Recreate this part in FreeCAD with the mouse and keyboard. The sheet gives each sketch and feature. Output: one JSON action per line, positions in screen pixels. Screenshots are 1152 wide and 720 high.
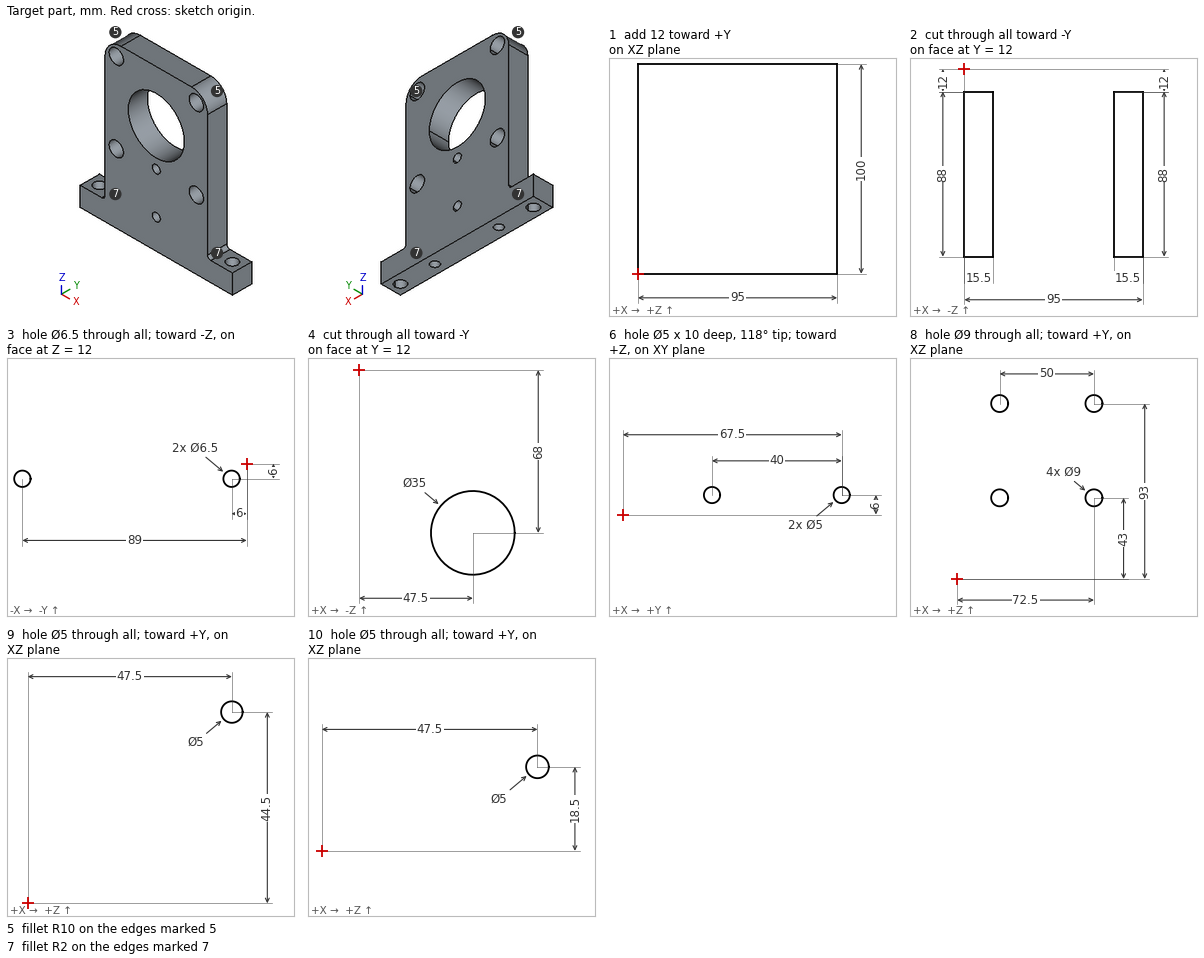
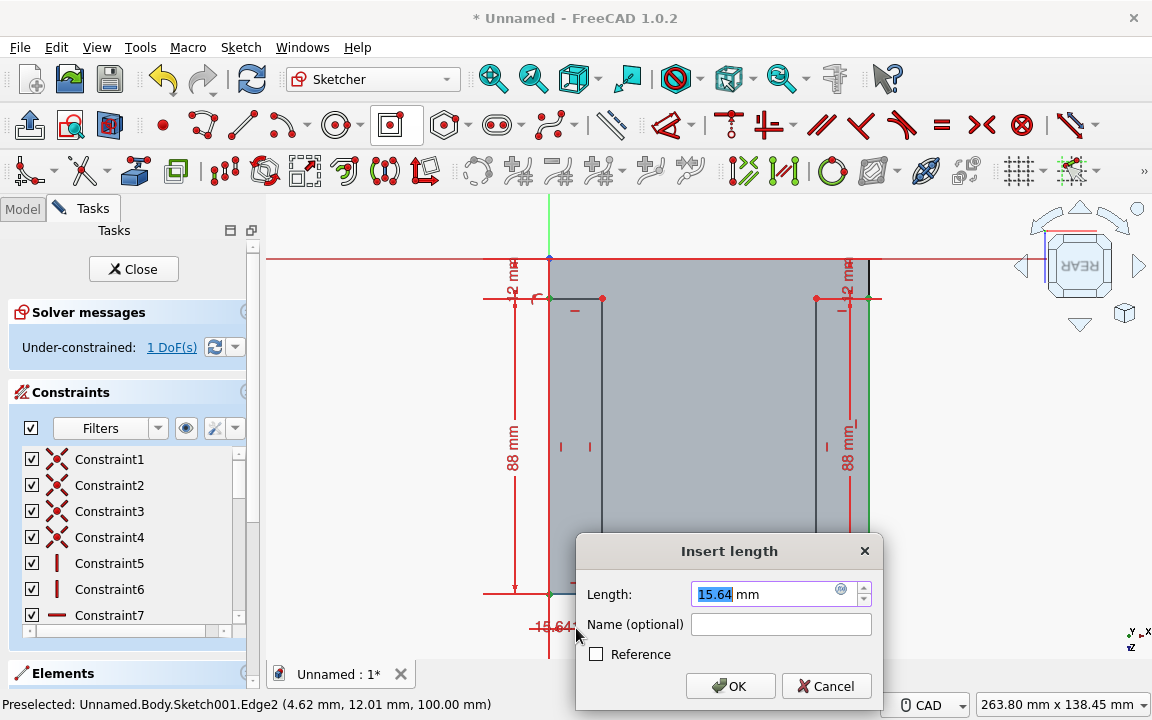
{"action": "type", "text": "15.5"}
{"action": "key", "text": "Return"}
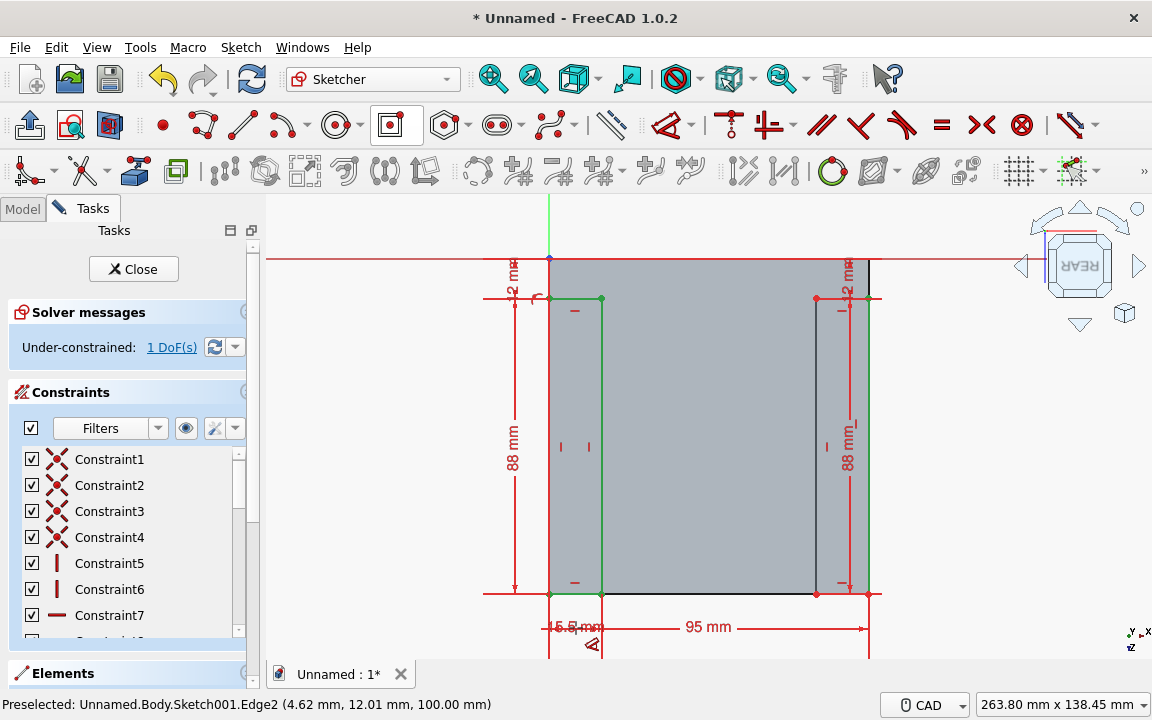
{"action": "left_click", "coordinate": [832, 594]}
{"action": "left_click", "coordinate": [842, 628]}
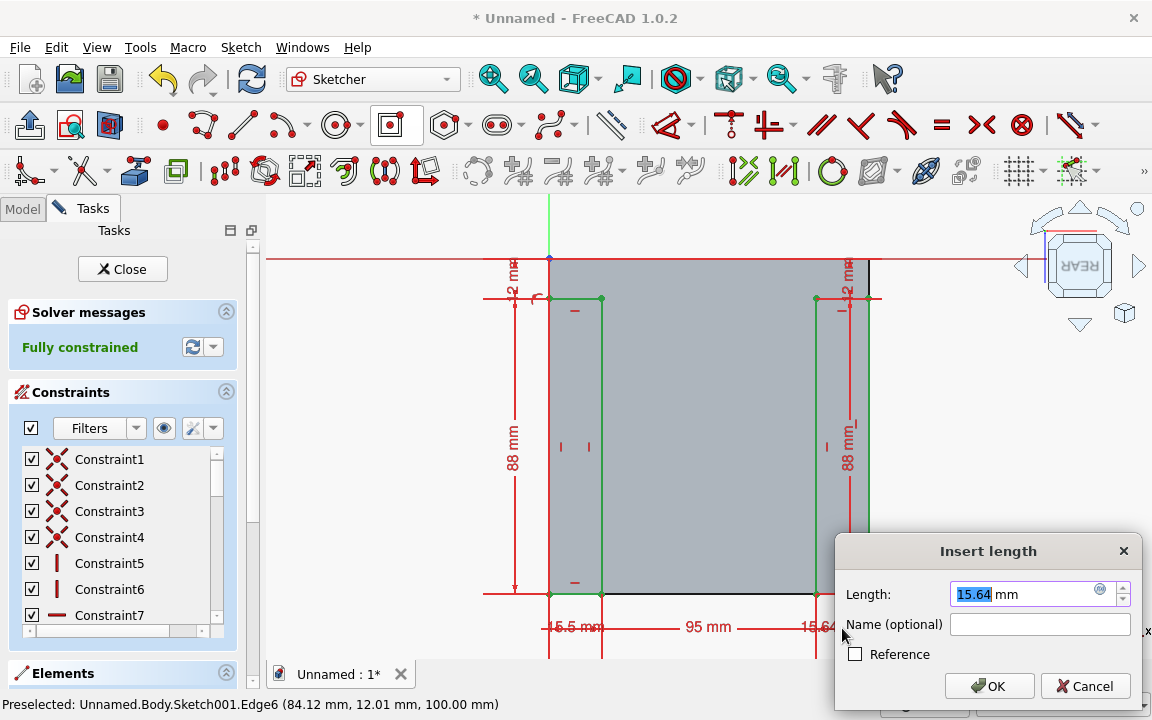
{"action": "type", "text": "15.5"}
{"action": "key", "text": "Return"}
{"action": "key", "text": "Escape"}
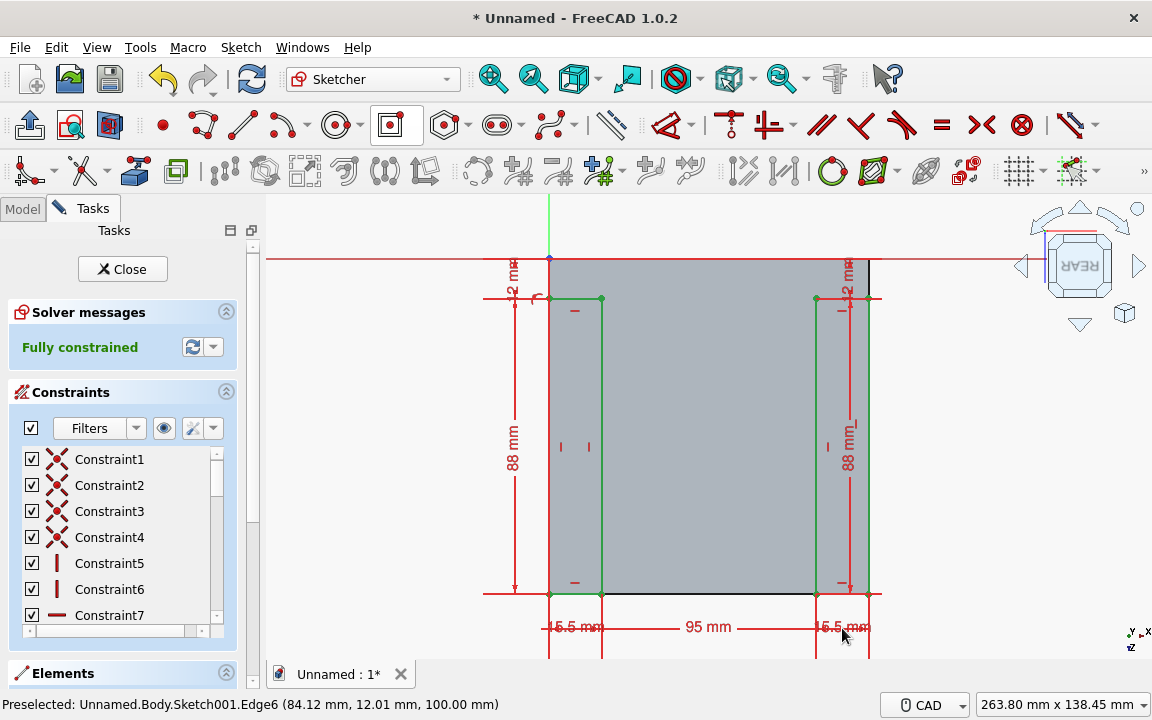
{"action": "left_click", "coordinate": [123, 269]}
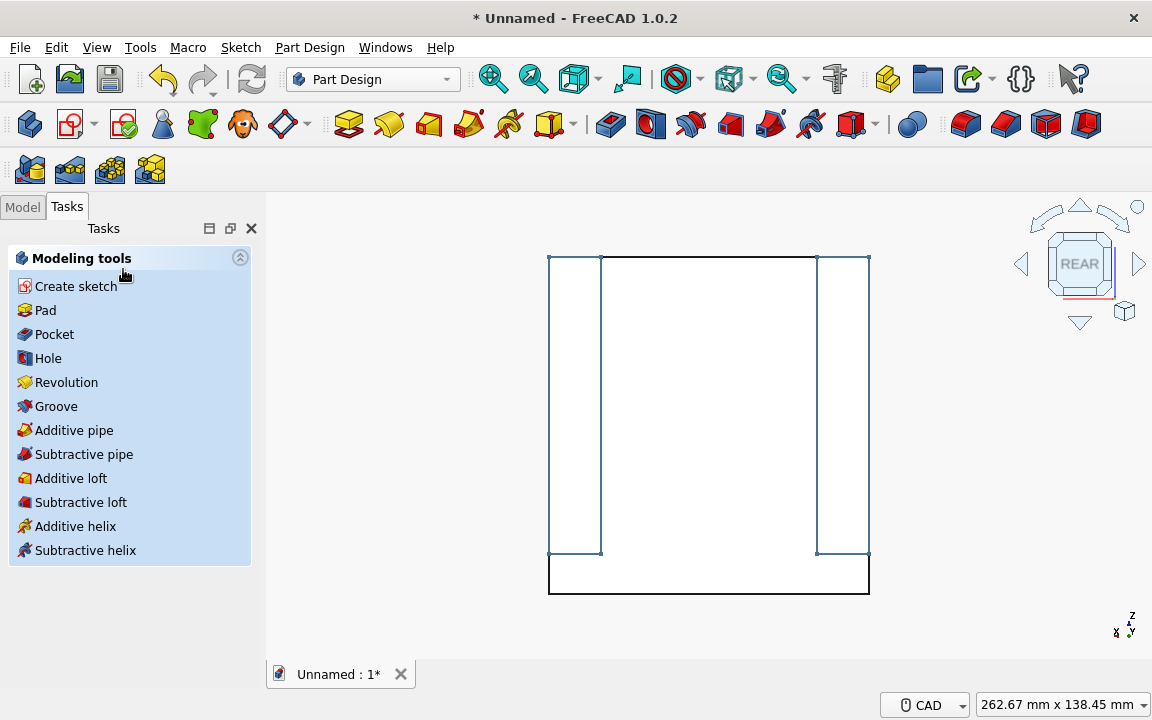
{"action": "left_click", "coordinate": [612, 124]}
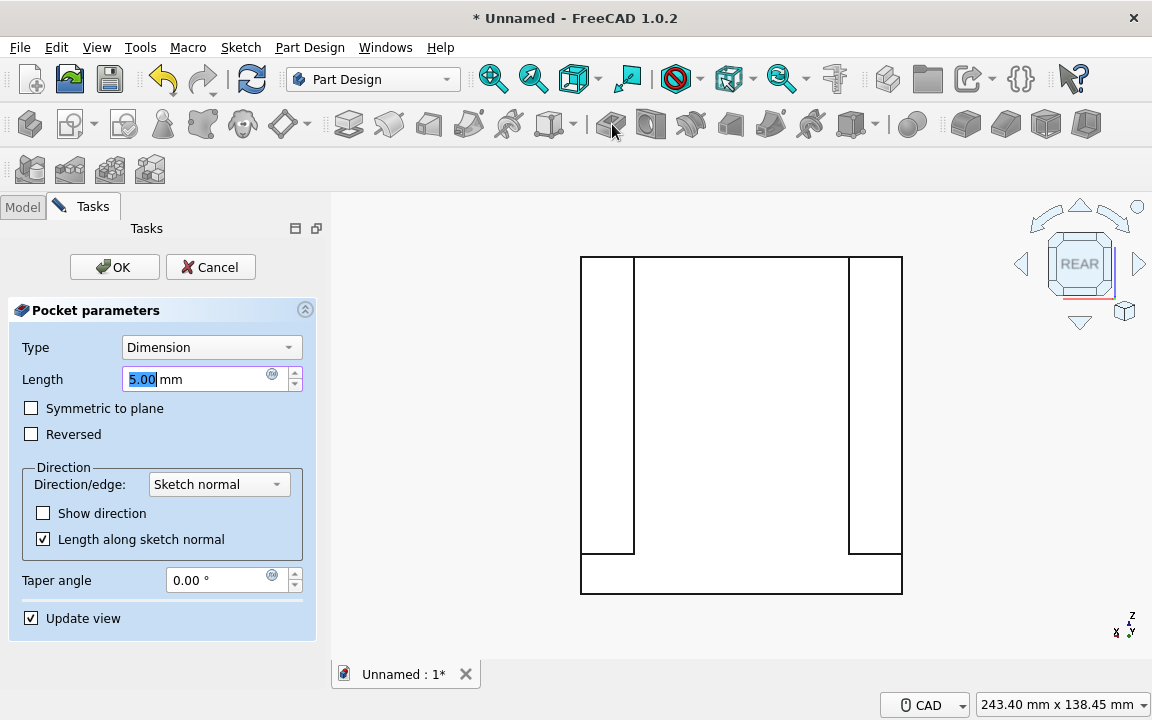
{"action": "left_click", "coordinate": [212, 348]}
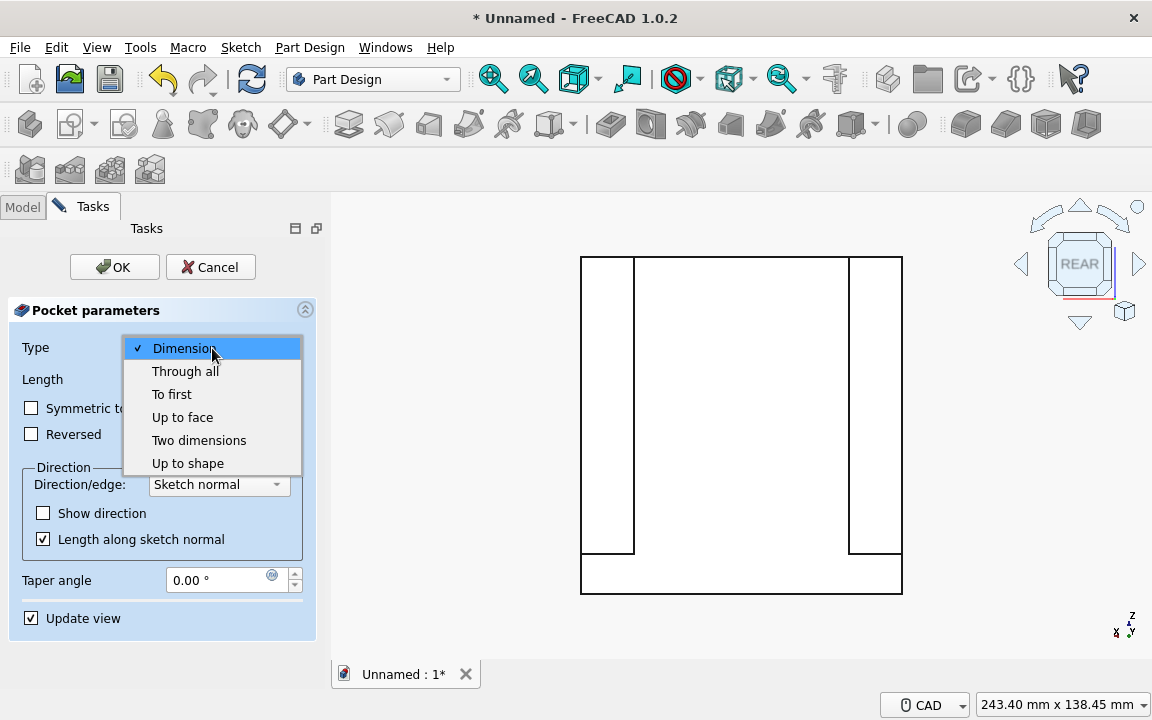
{"action": "left_click", "coordinate": [212, 372]}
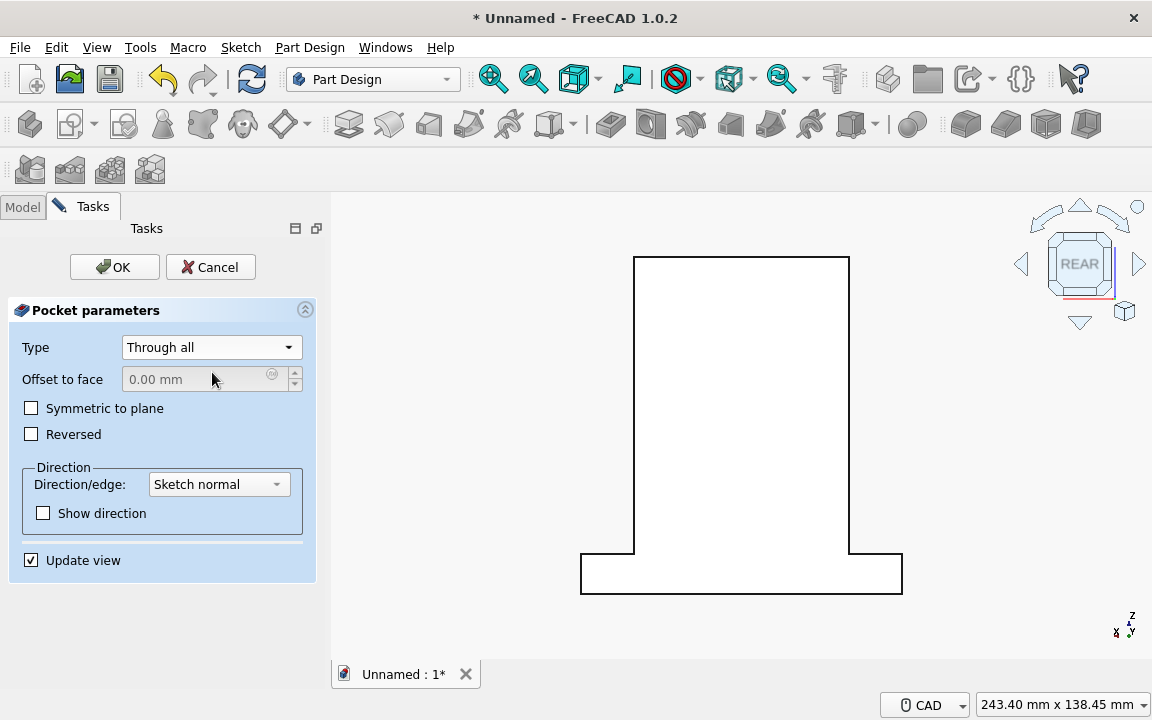
{"action": "left_click", "coordinate": [115, 267]}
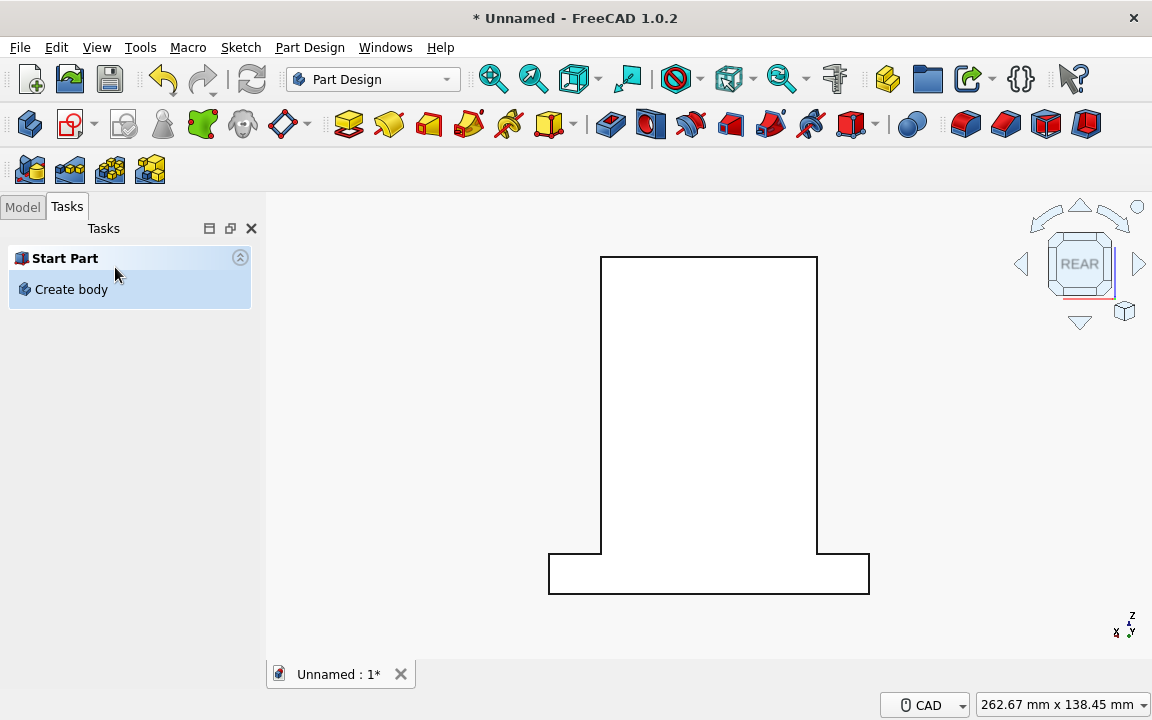
{"action": "key", "text": "0"}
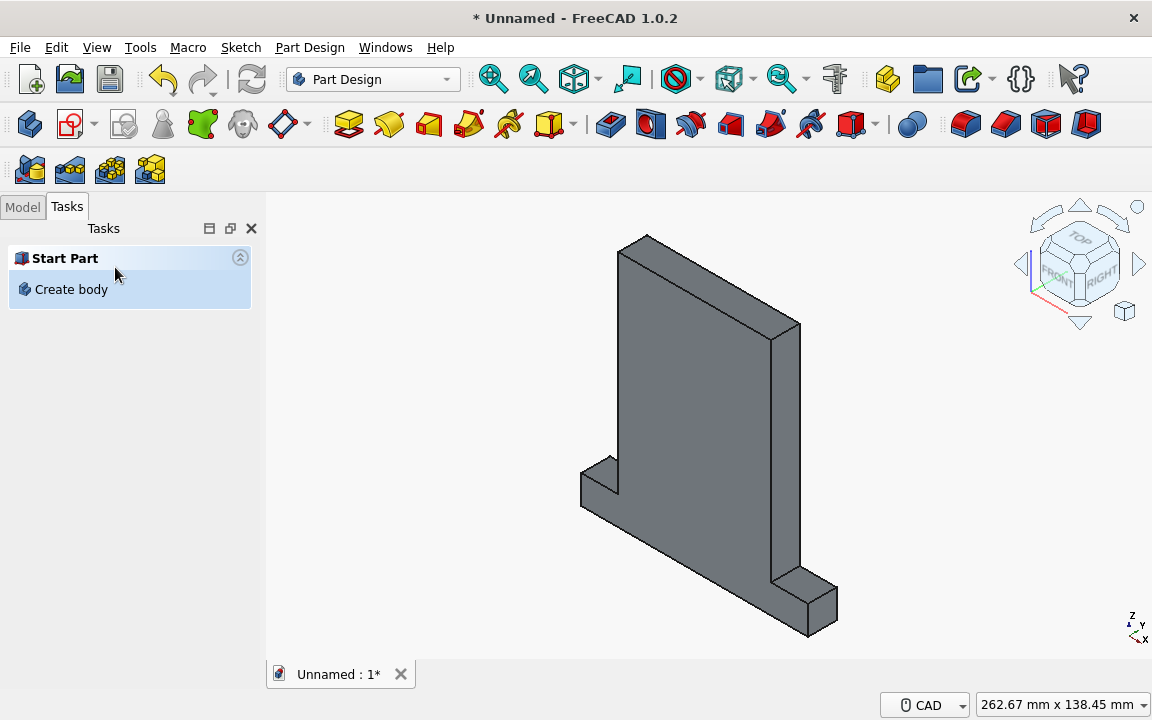
{"action": "left_click", "coordinate": [609, 471]}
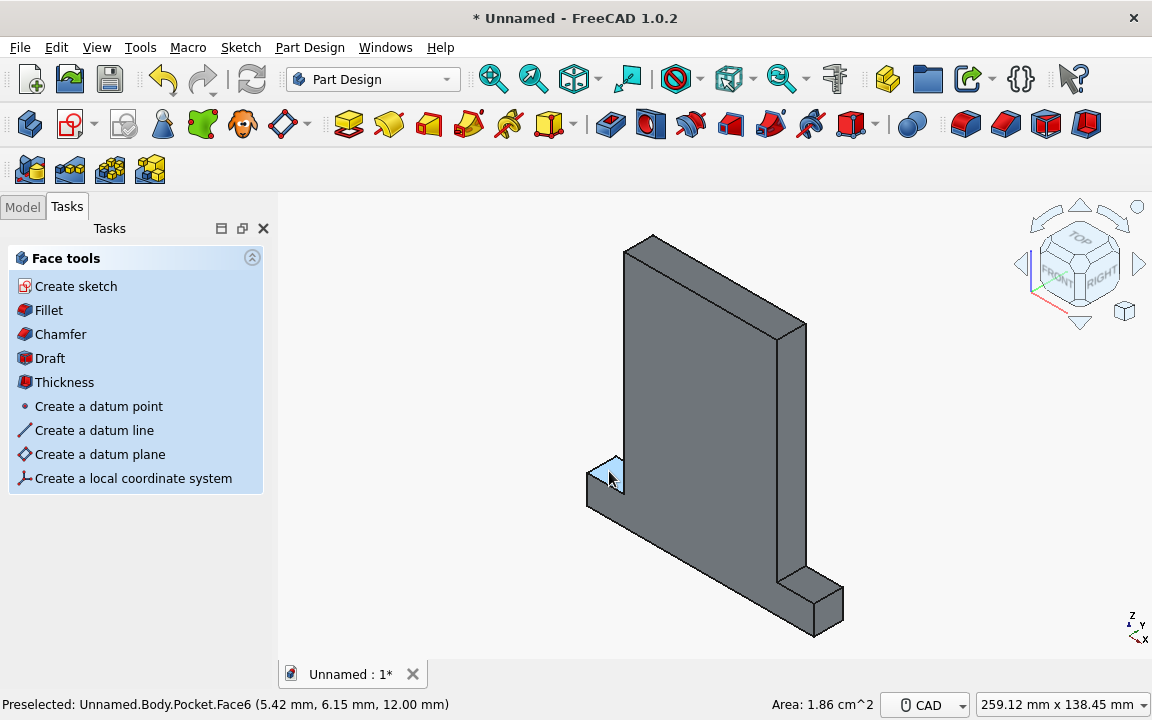
{"action": "left_click", "coordinate": [70, 124]}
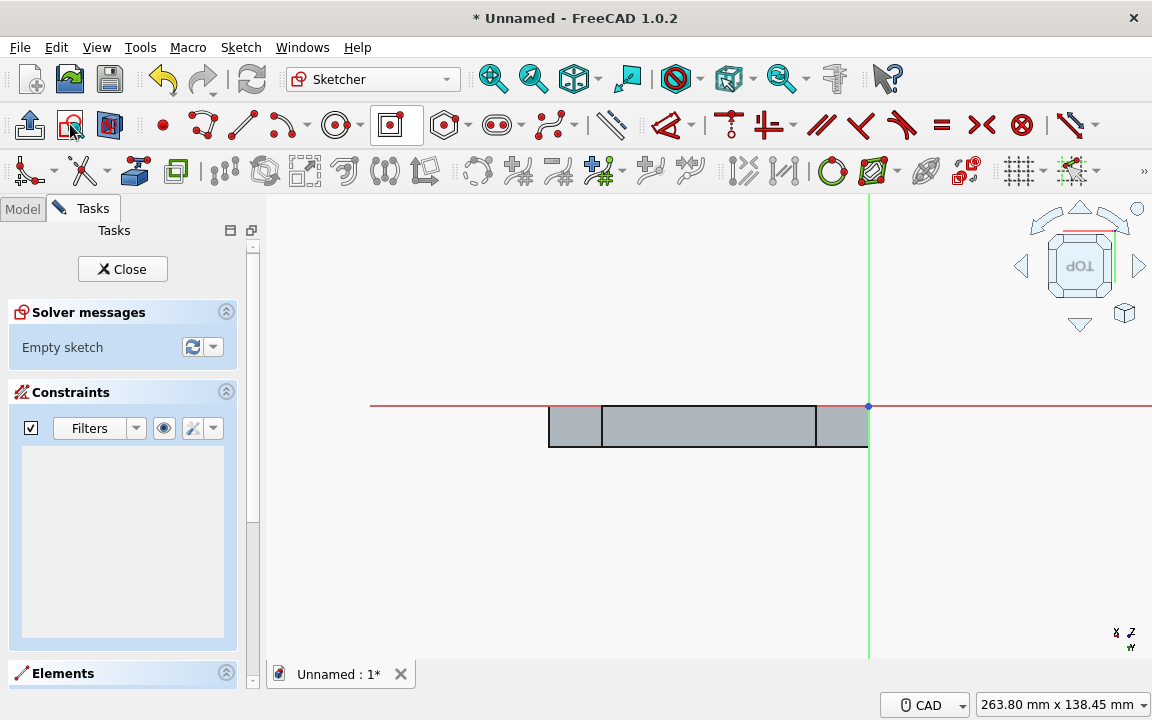
{"action": "left_click", "coordinate": [110, 126]}